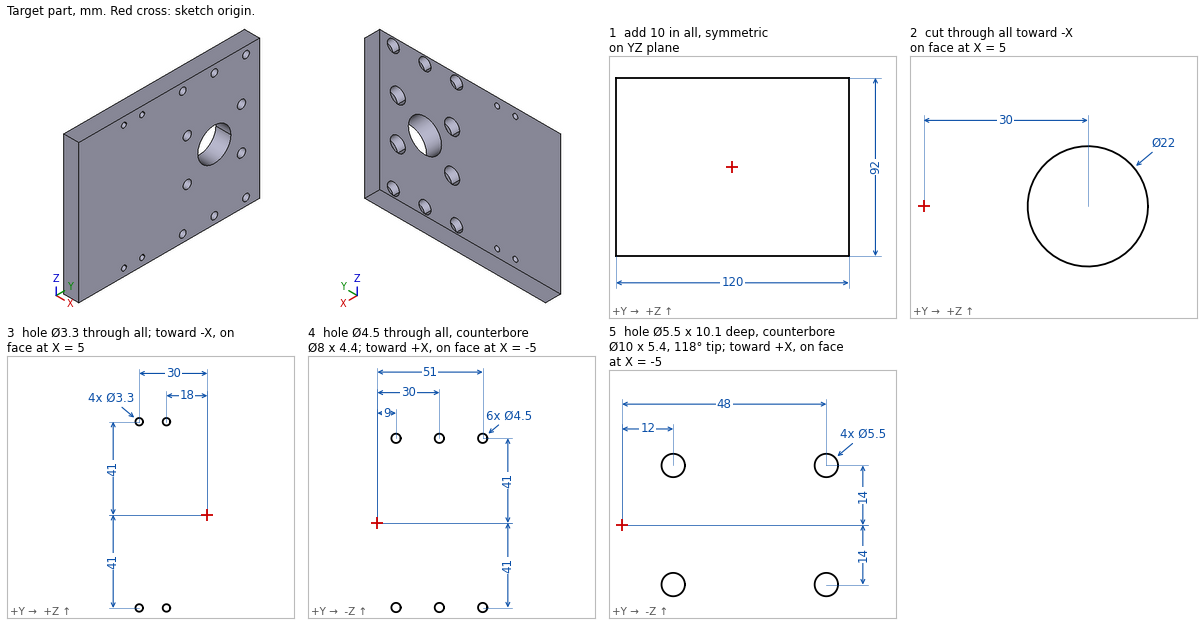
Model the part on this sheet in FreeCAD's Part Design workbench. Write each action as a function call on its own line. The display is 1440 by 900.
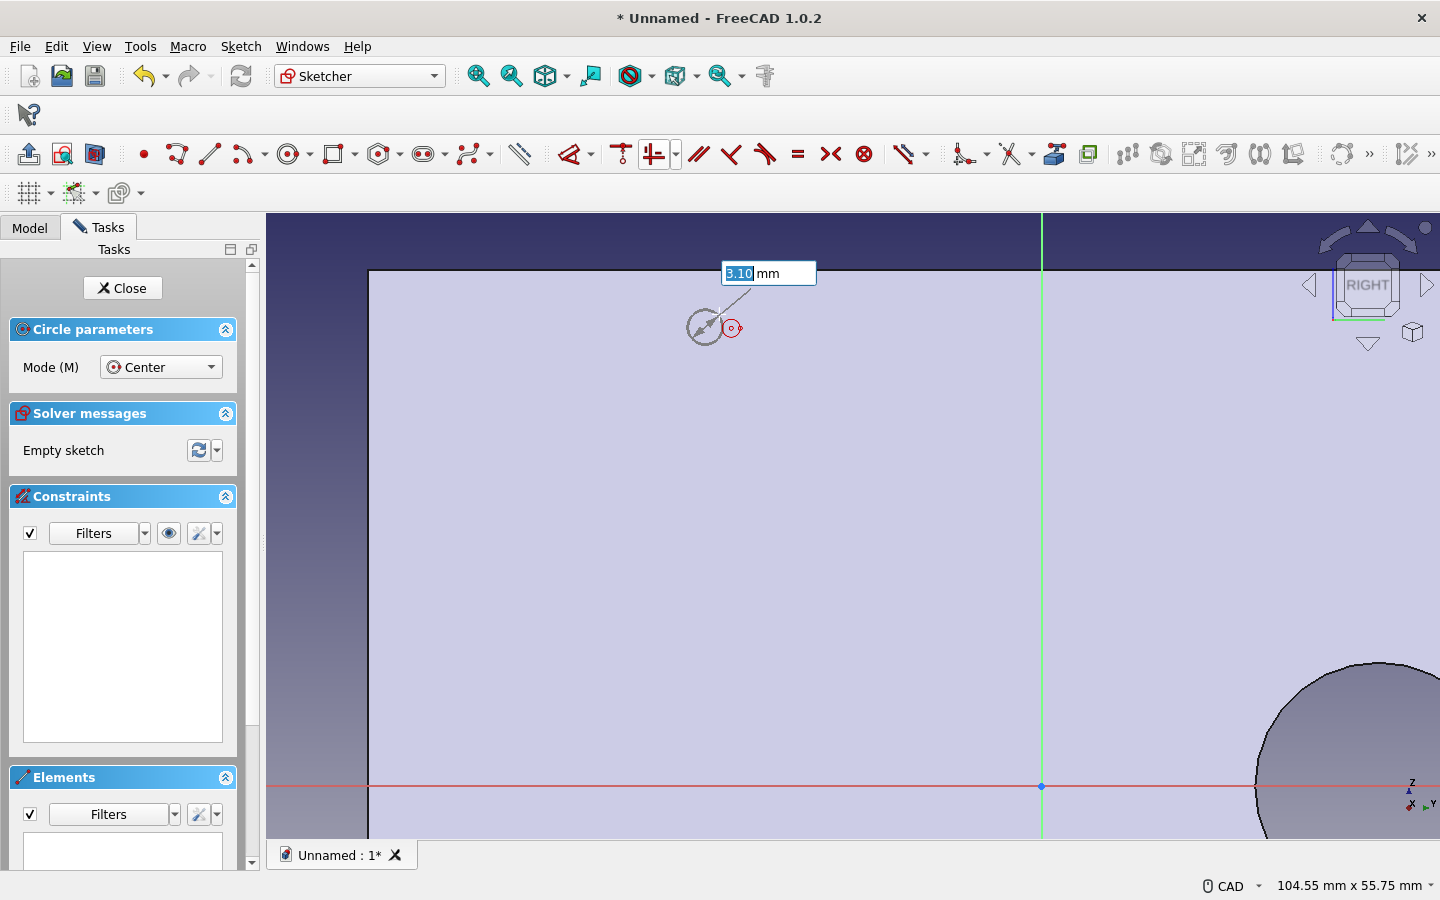
click(718, 313)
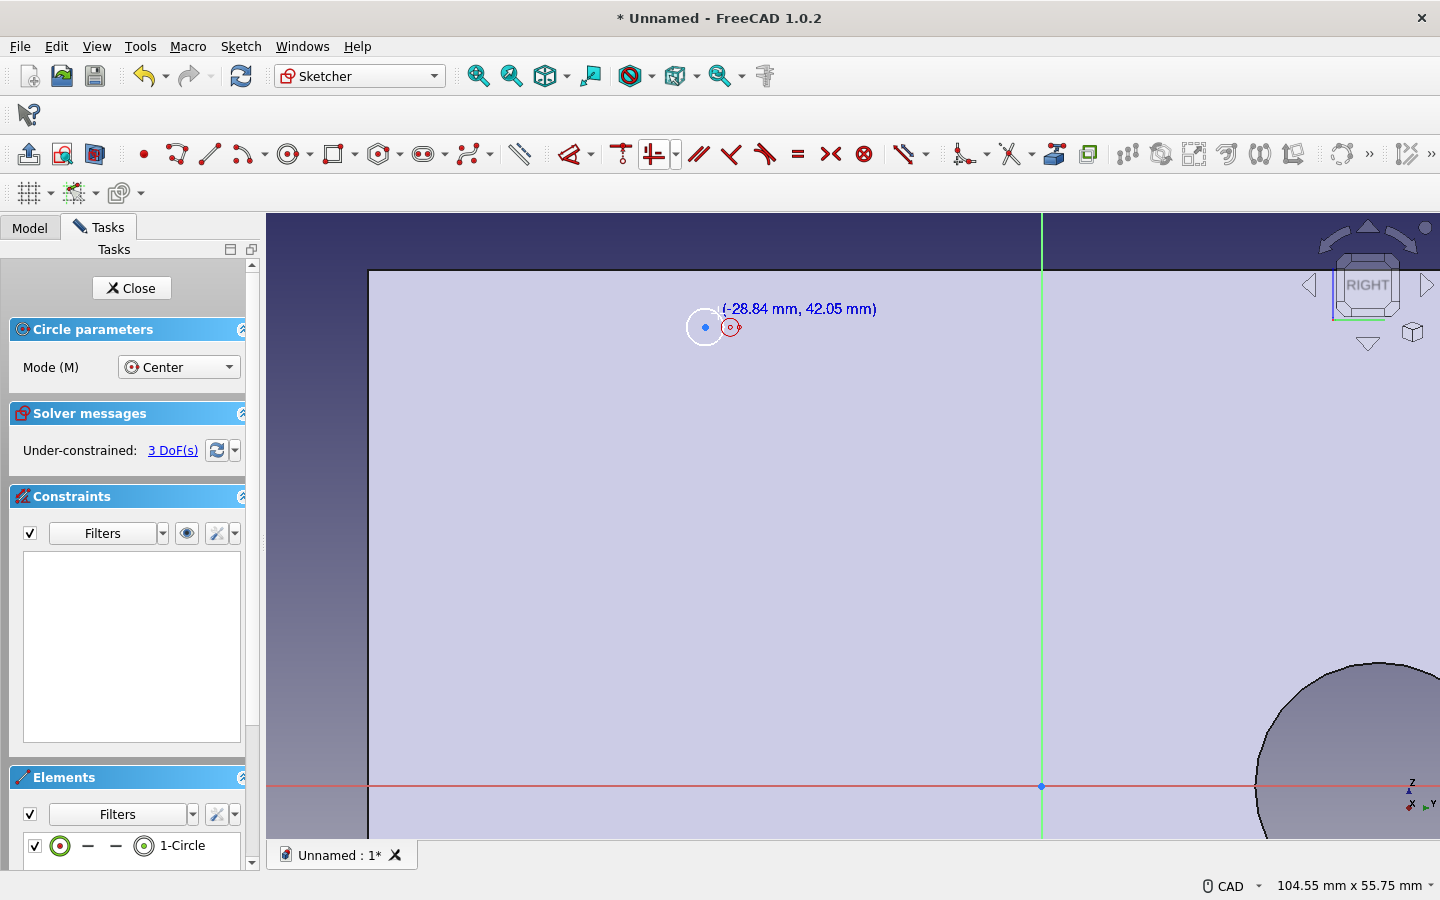
scroll(840, 326, up, 2)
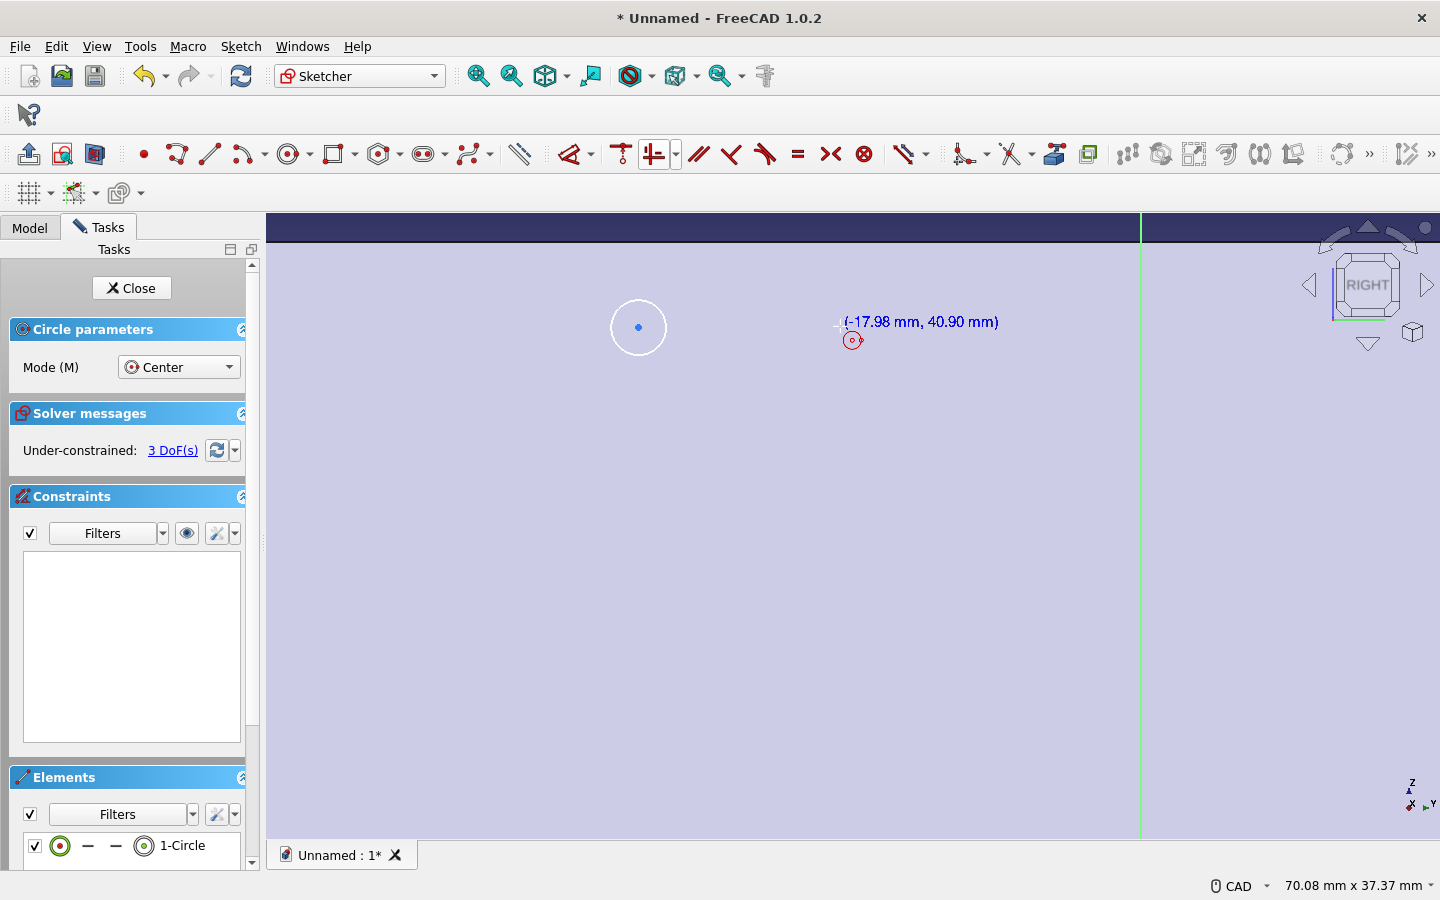
scroll(745, 316, down, 6)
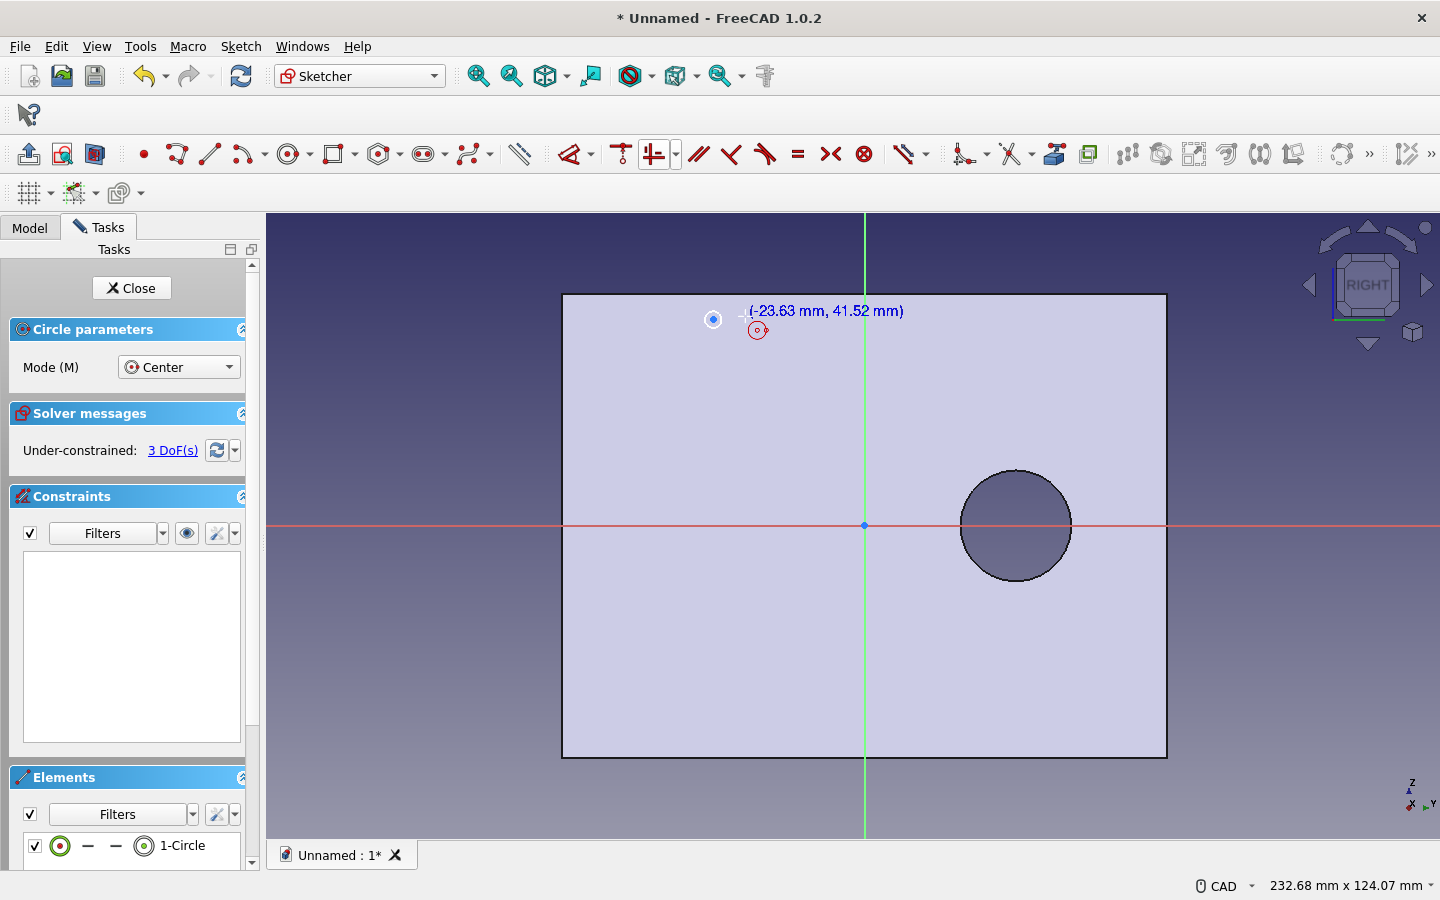
click(774, 319)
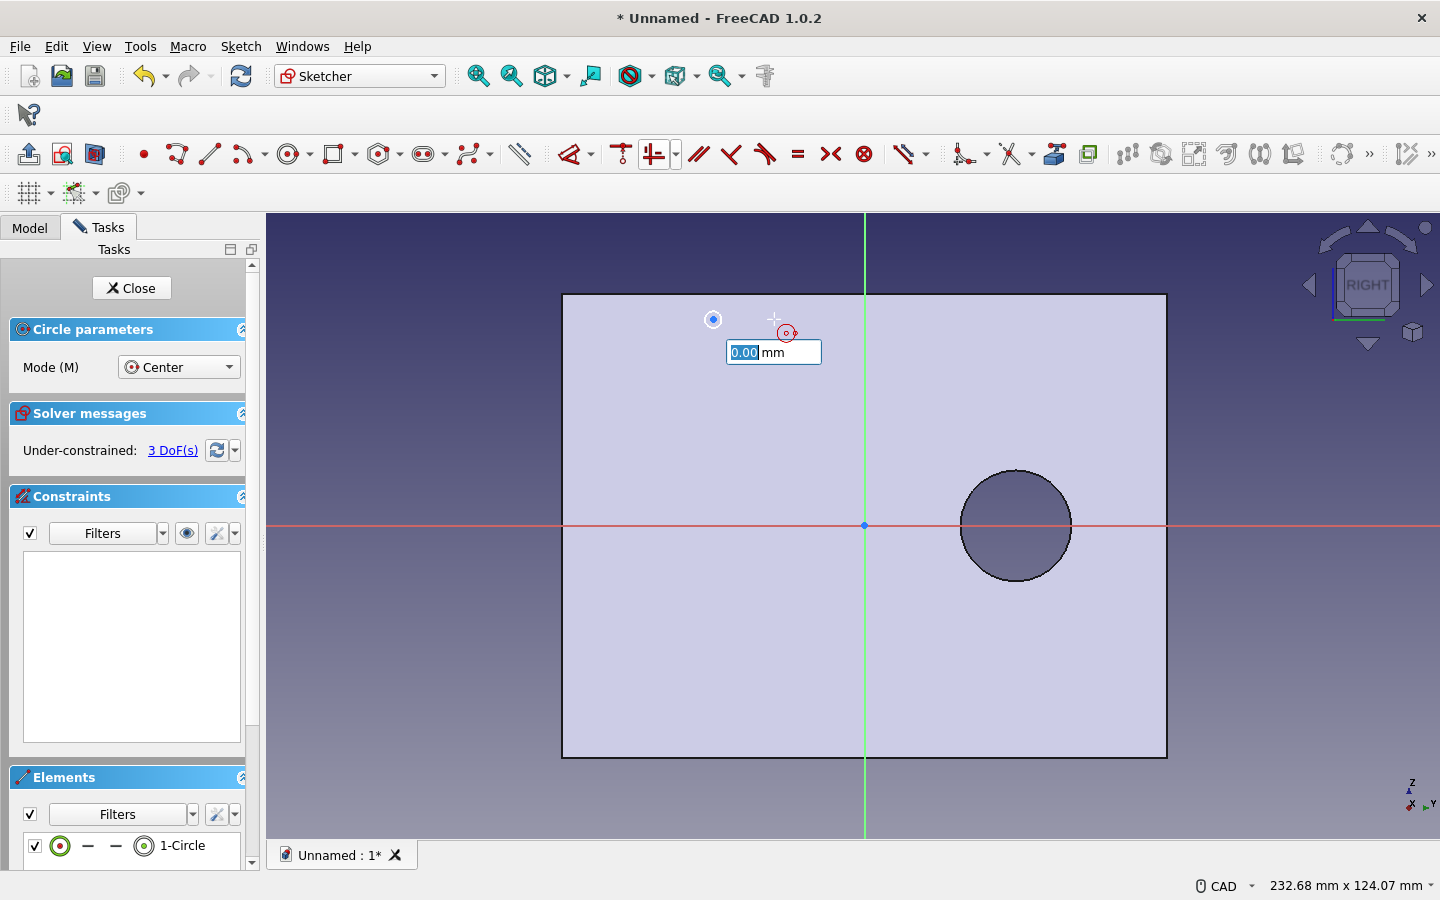
scroll(780, 313, up, 4)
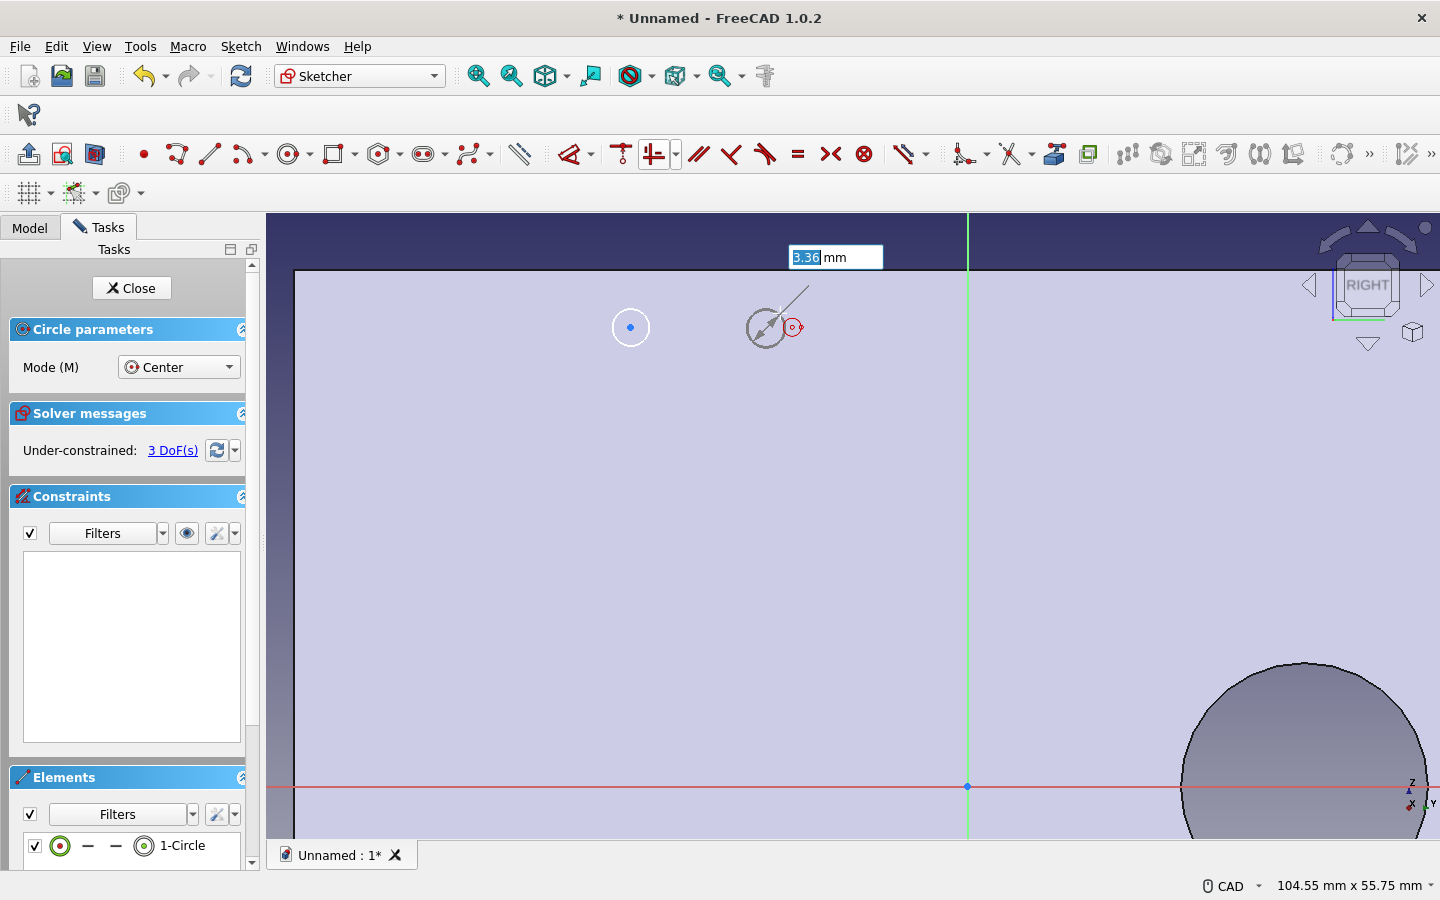
click(779, 313)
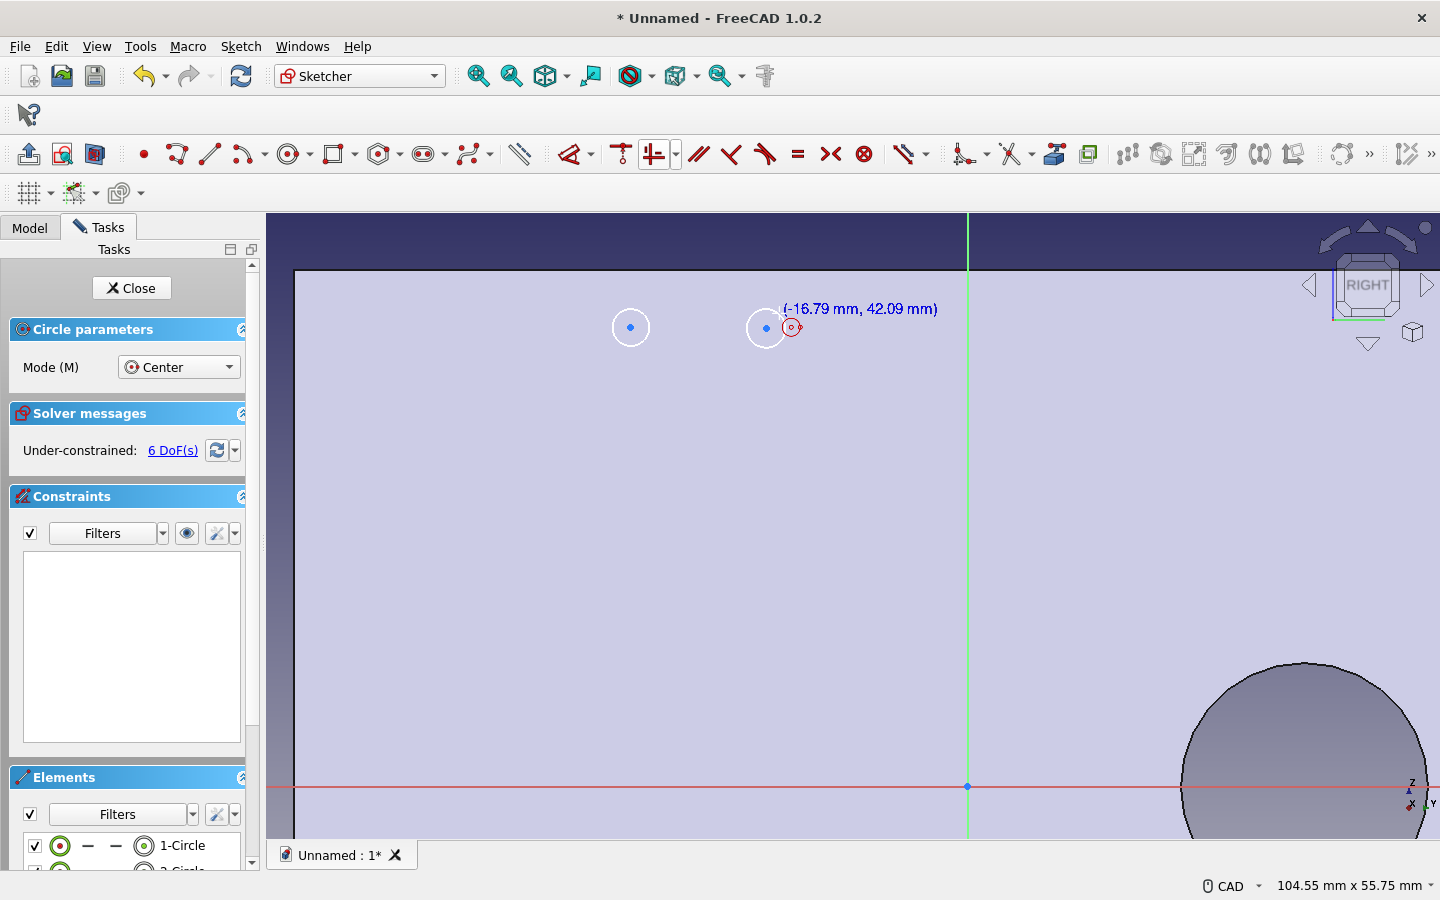
scroll(780, 313, down, 4)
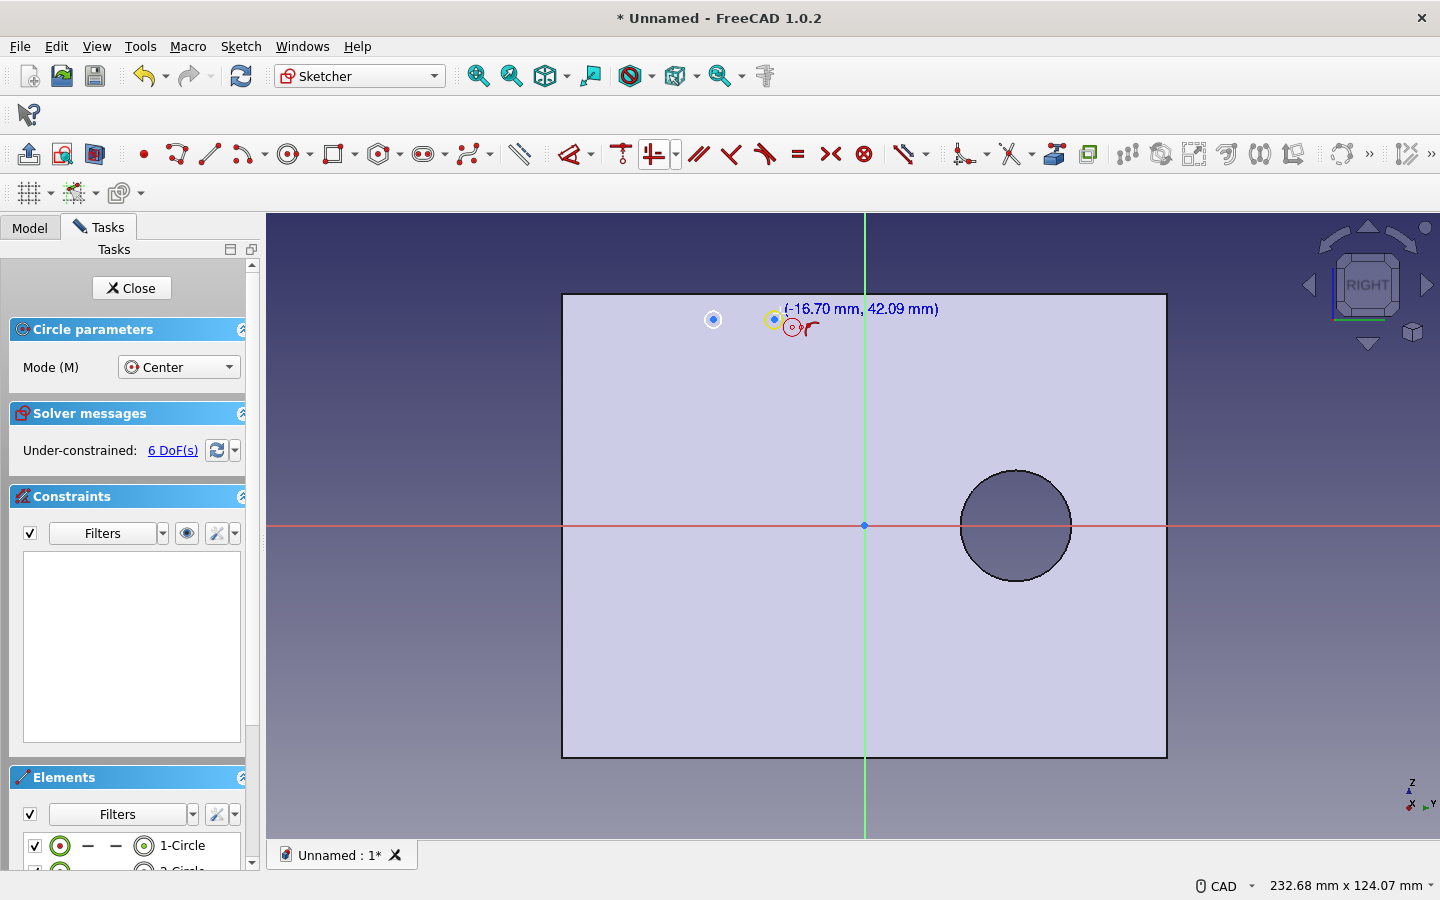
scroll(713, 733, up, 6)